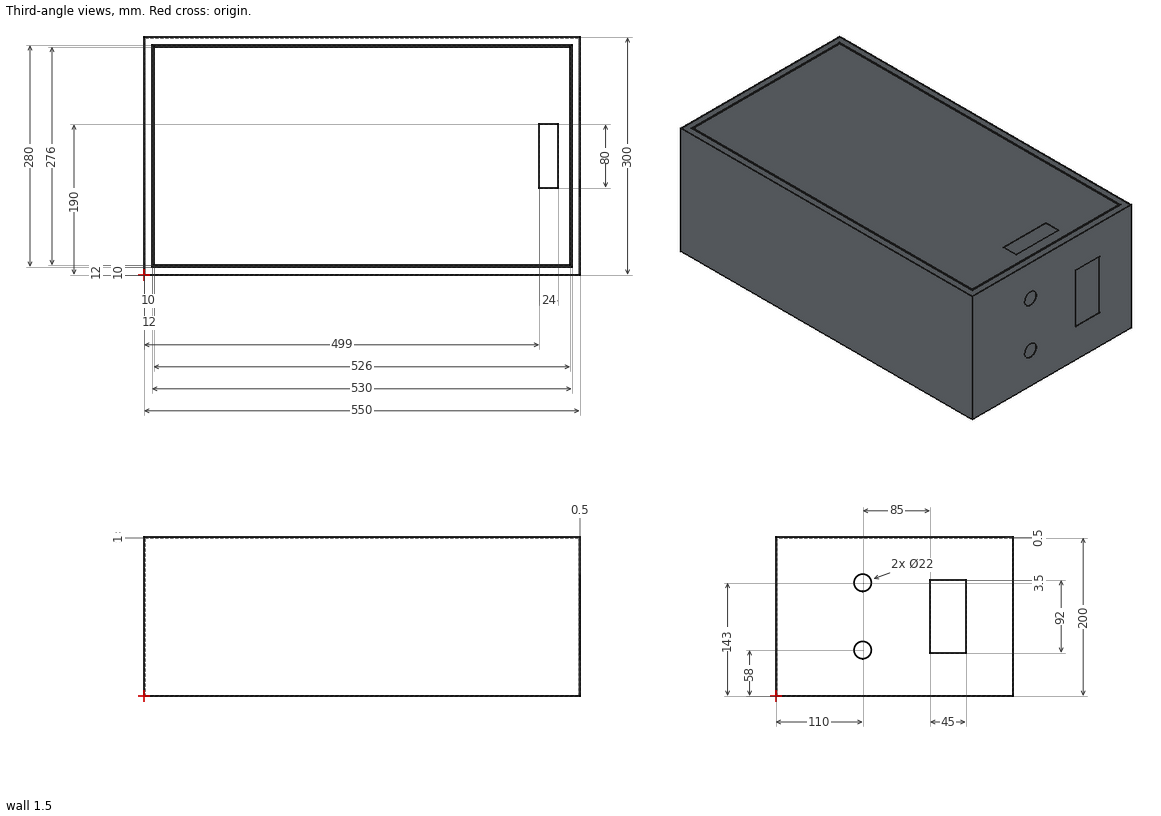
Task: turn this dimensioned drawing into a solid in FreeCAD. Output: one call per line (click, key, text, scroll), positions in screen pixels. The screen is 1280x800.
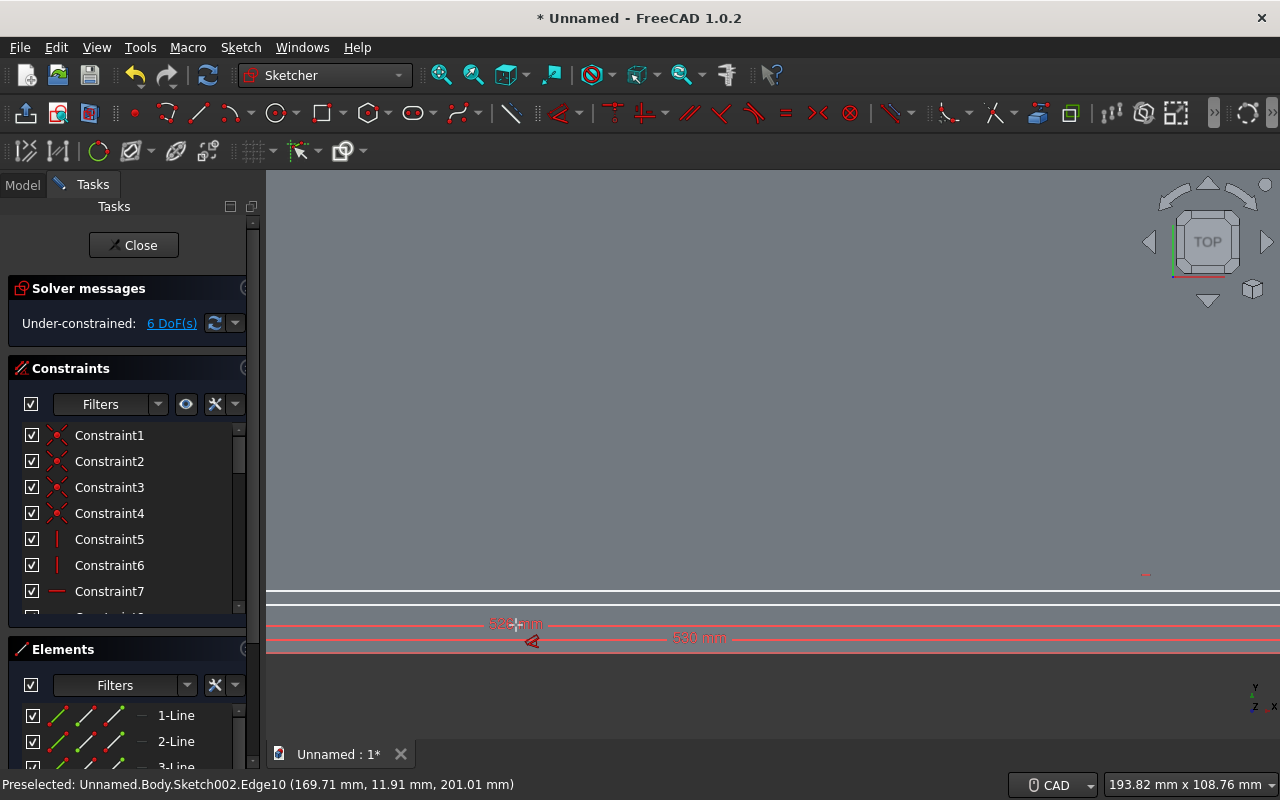
scroll(599, 596, down, 8)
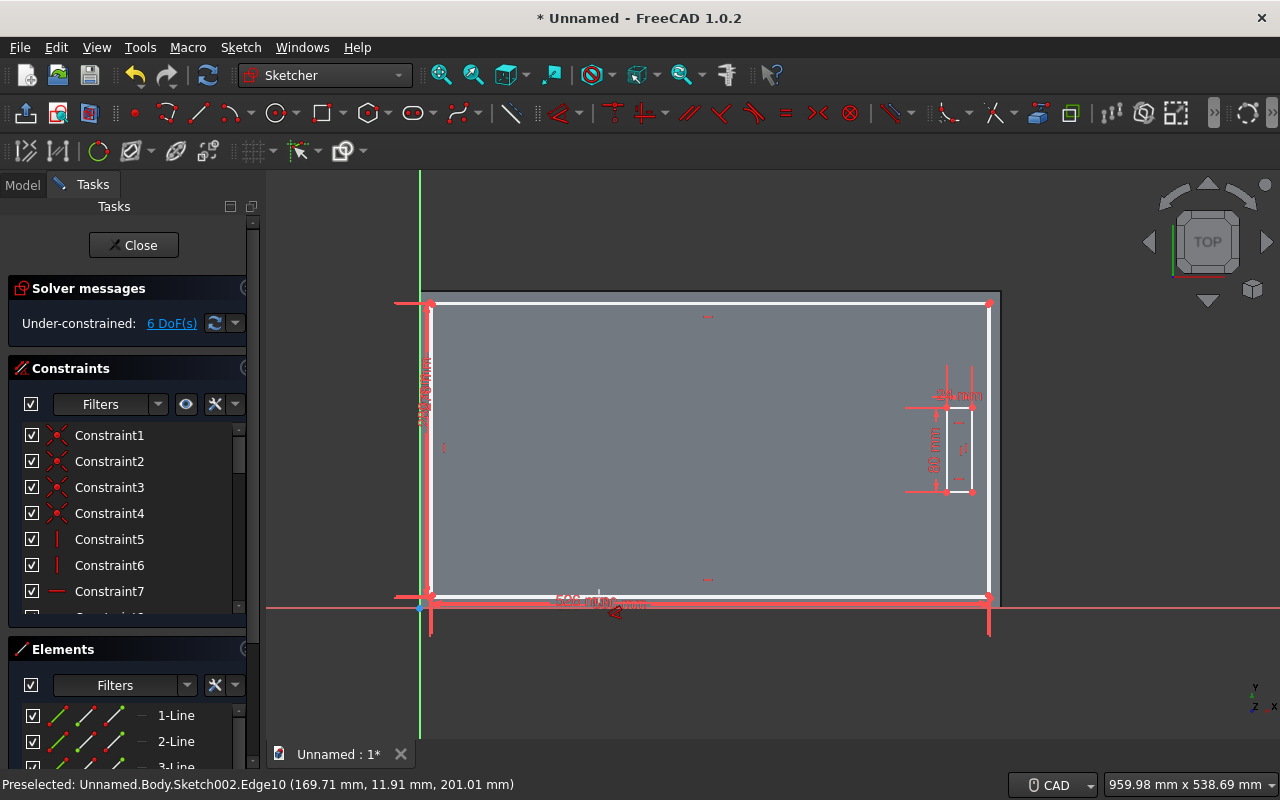
scroll(430, 303, up, 8)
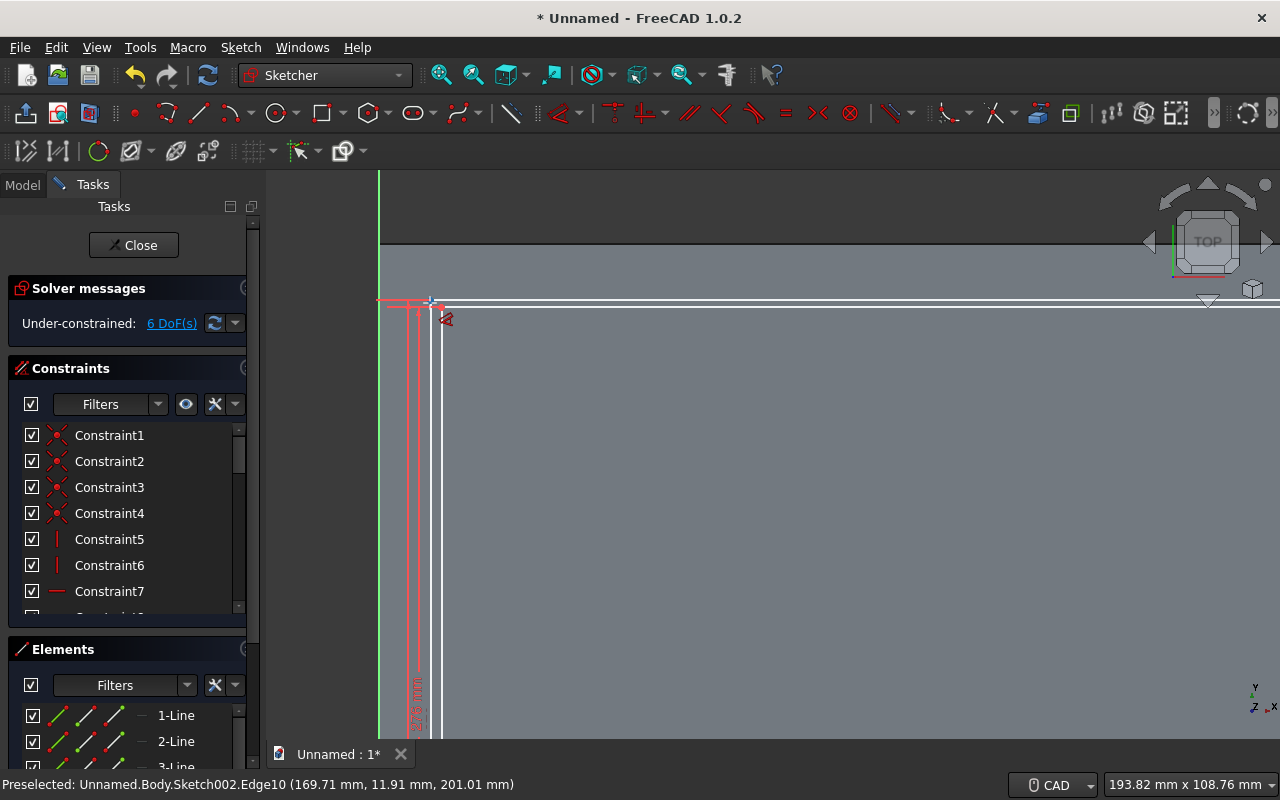
click(431, 300)
click(405, 266)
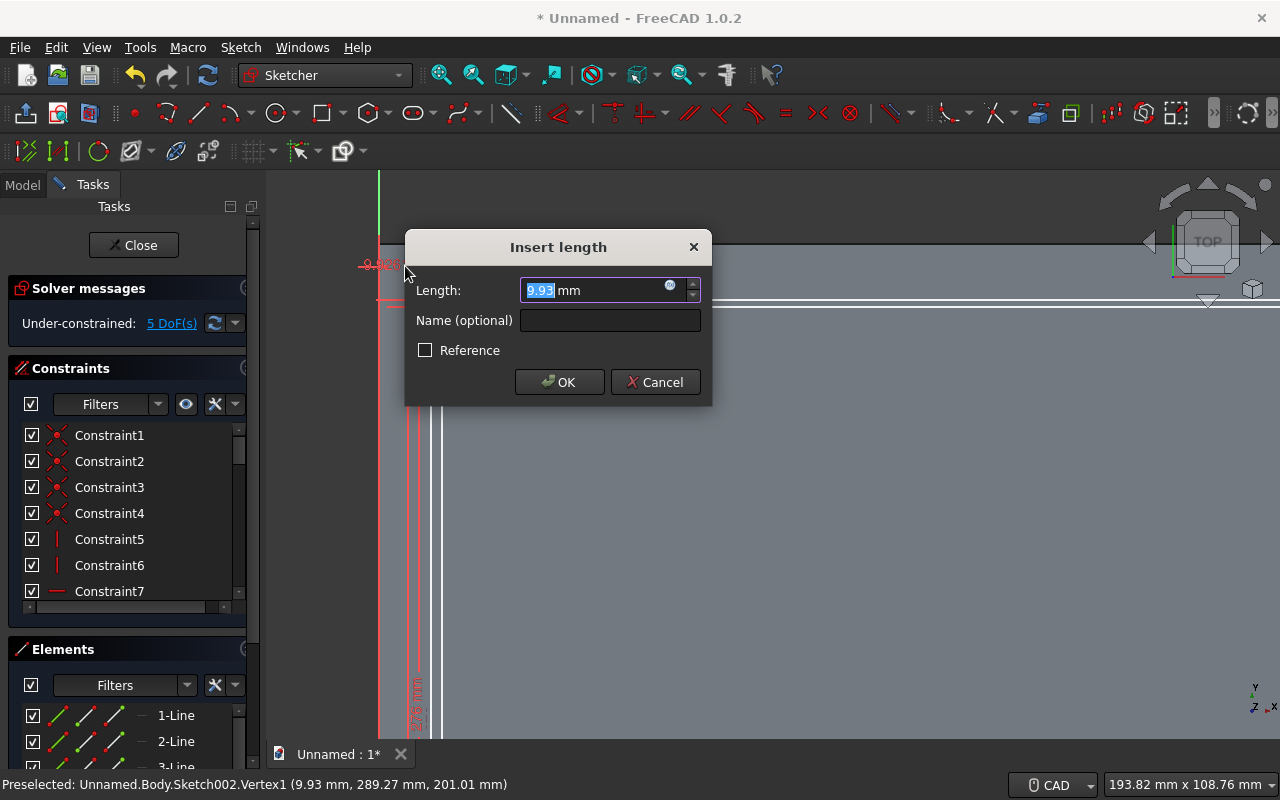
text(10)
key(Return)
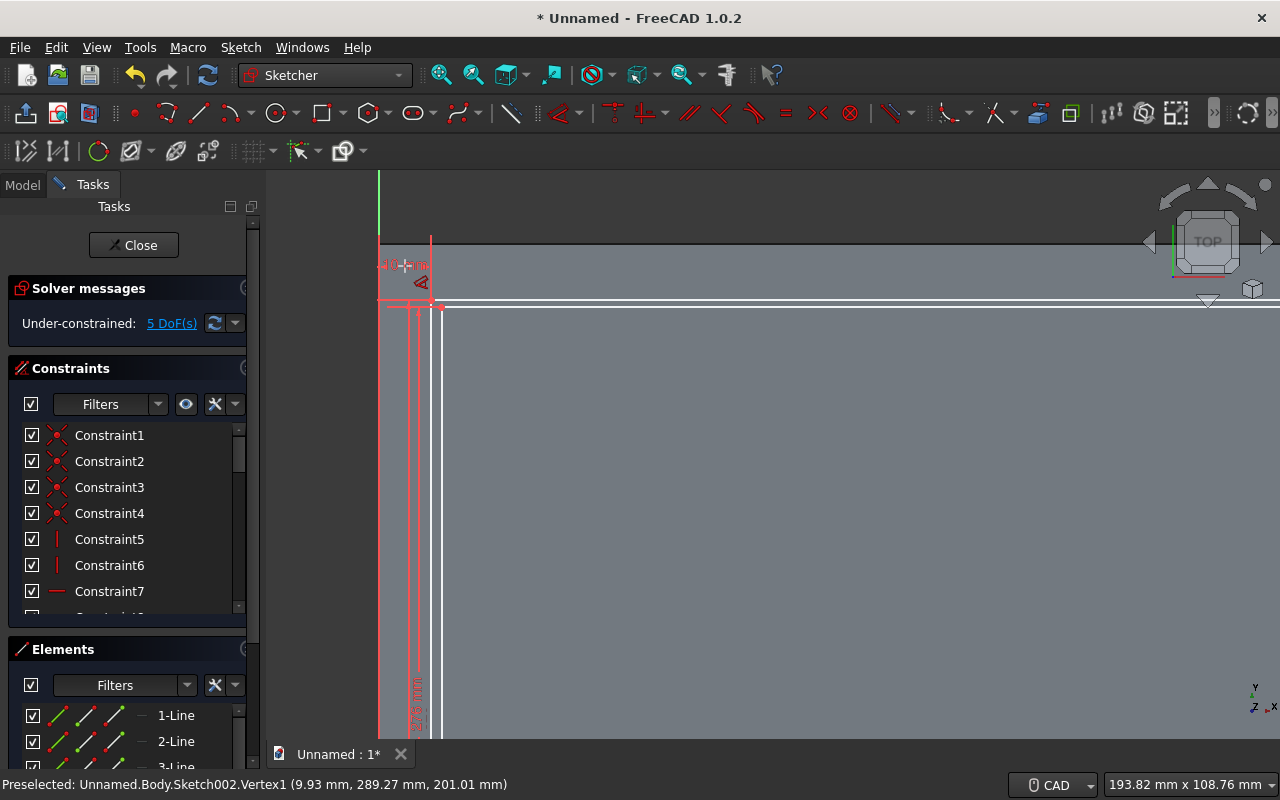
scroll(430, 303, down, 8)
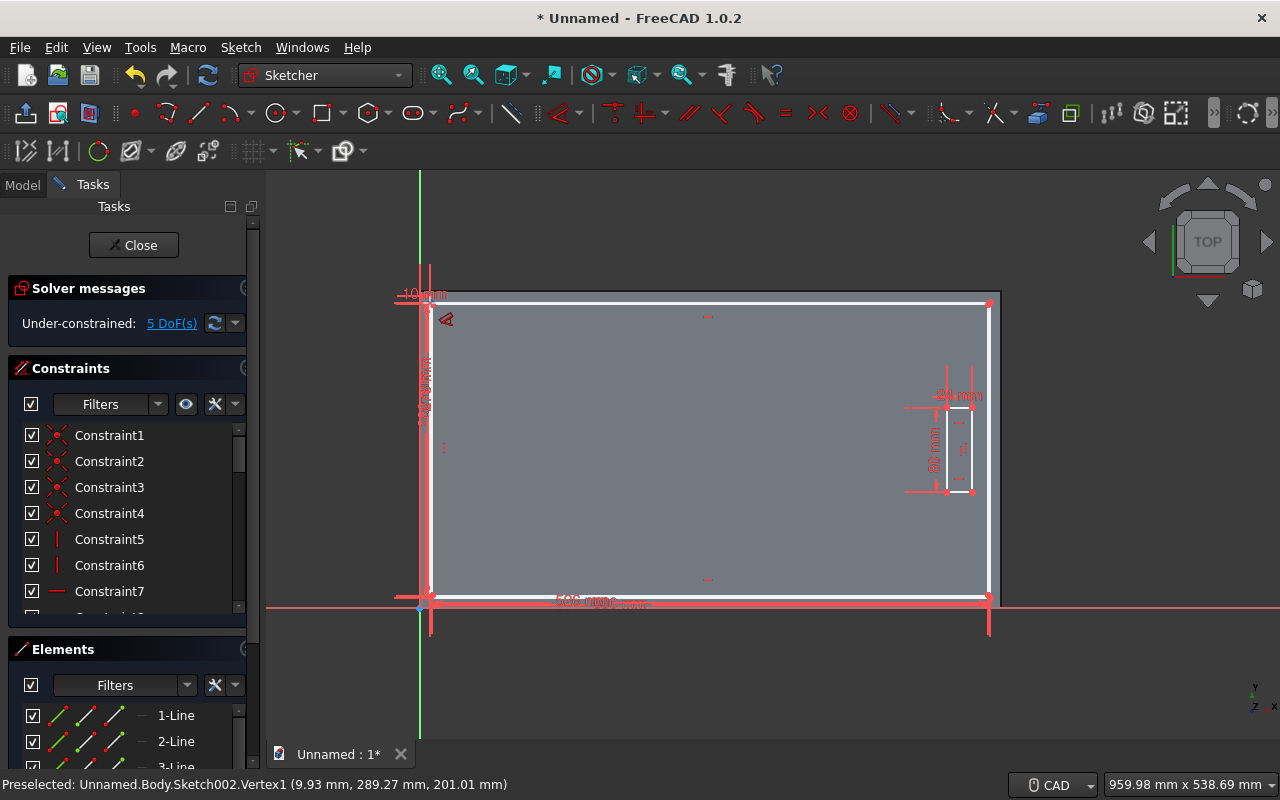
scroll(430, 598, up, 7)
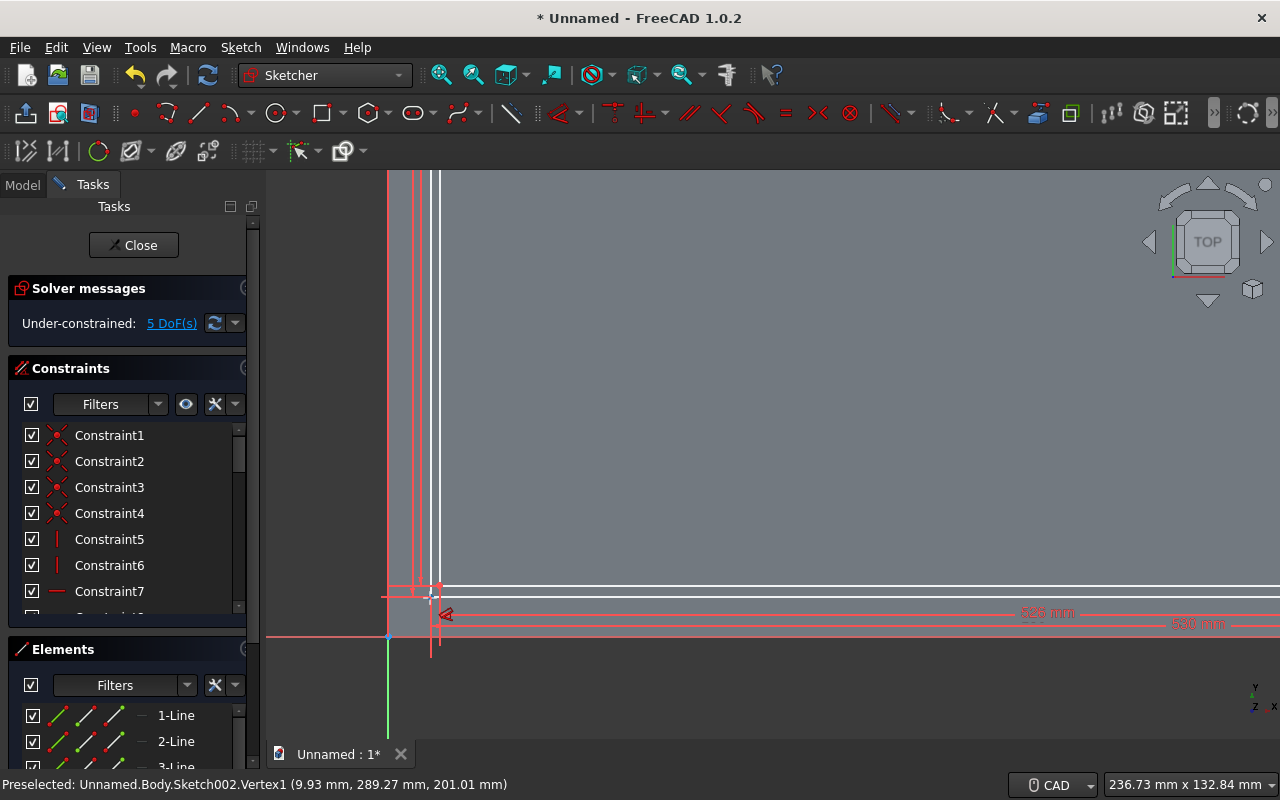
click(431, 597)
click(354, 617)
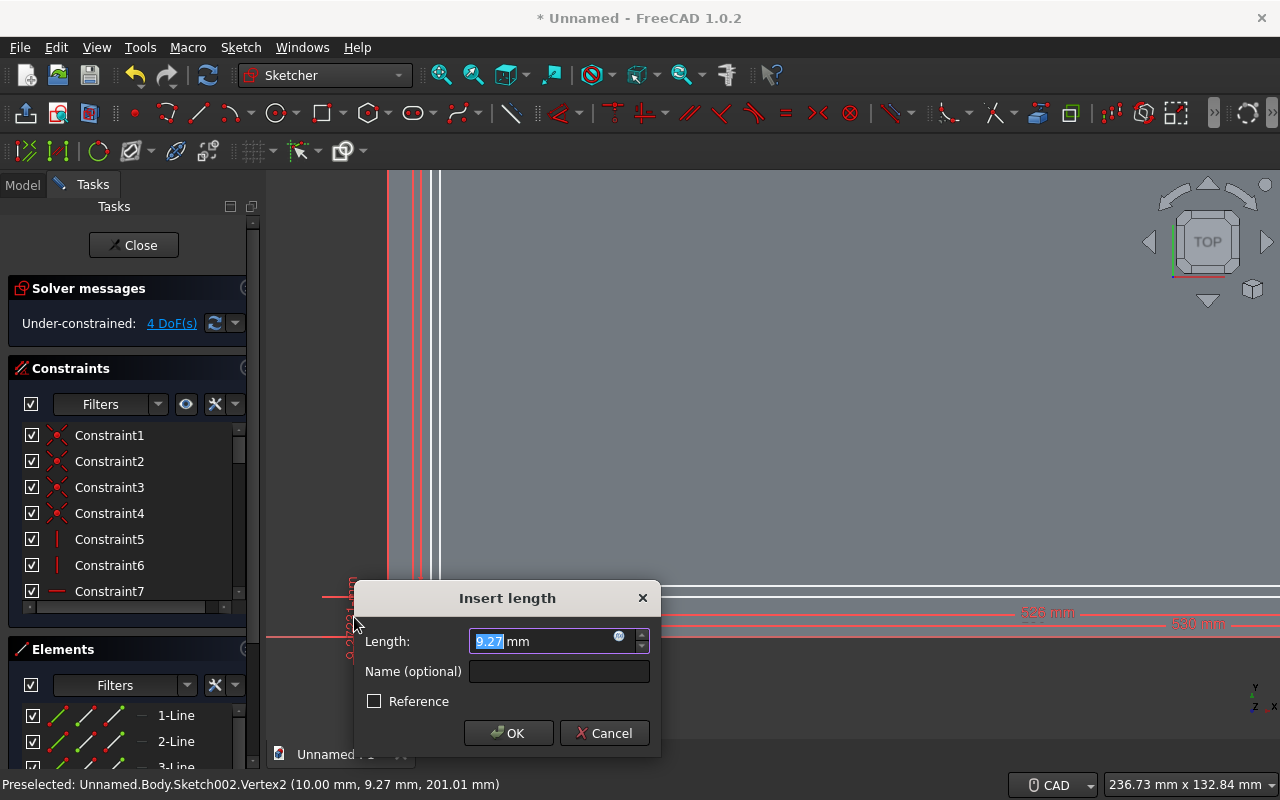
text(10)
key(Return)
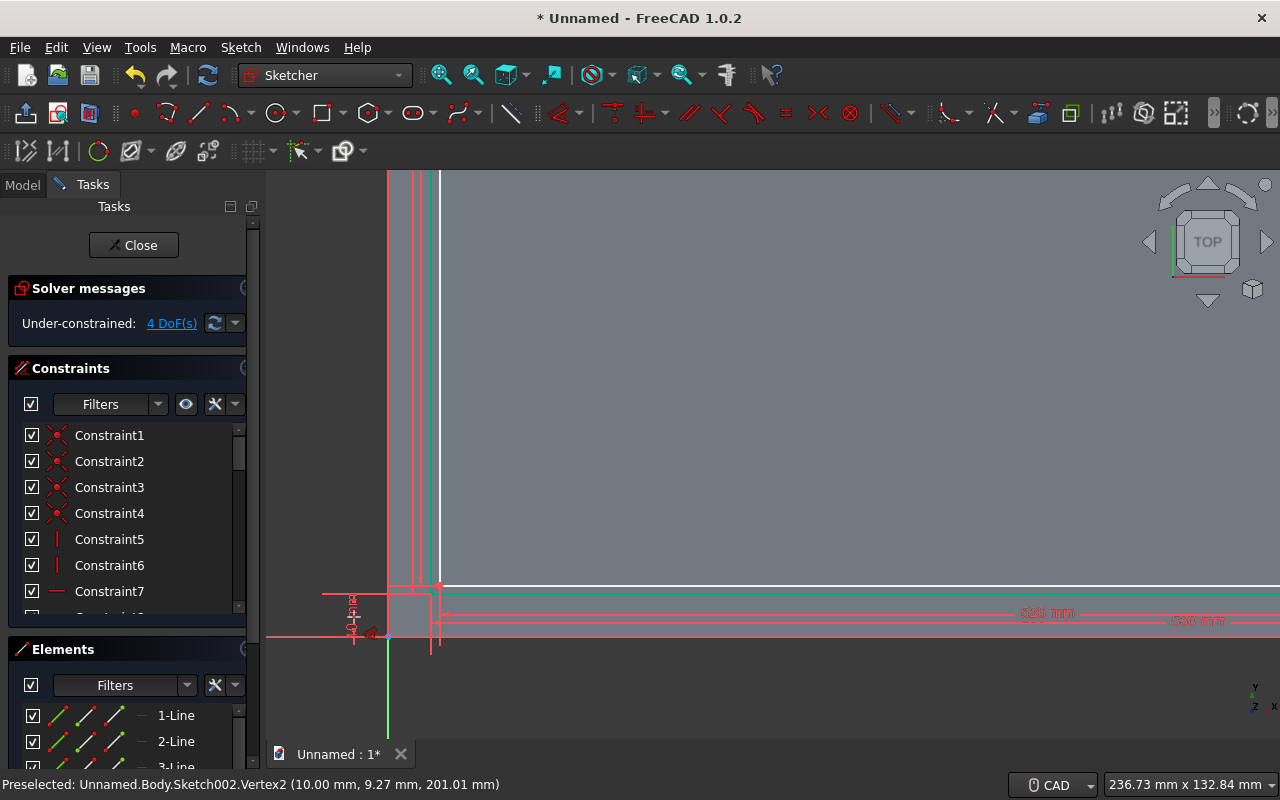
scroll(430, 598, down, 7)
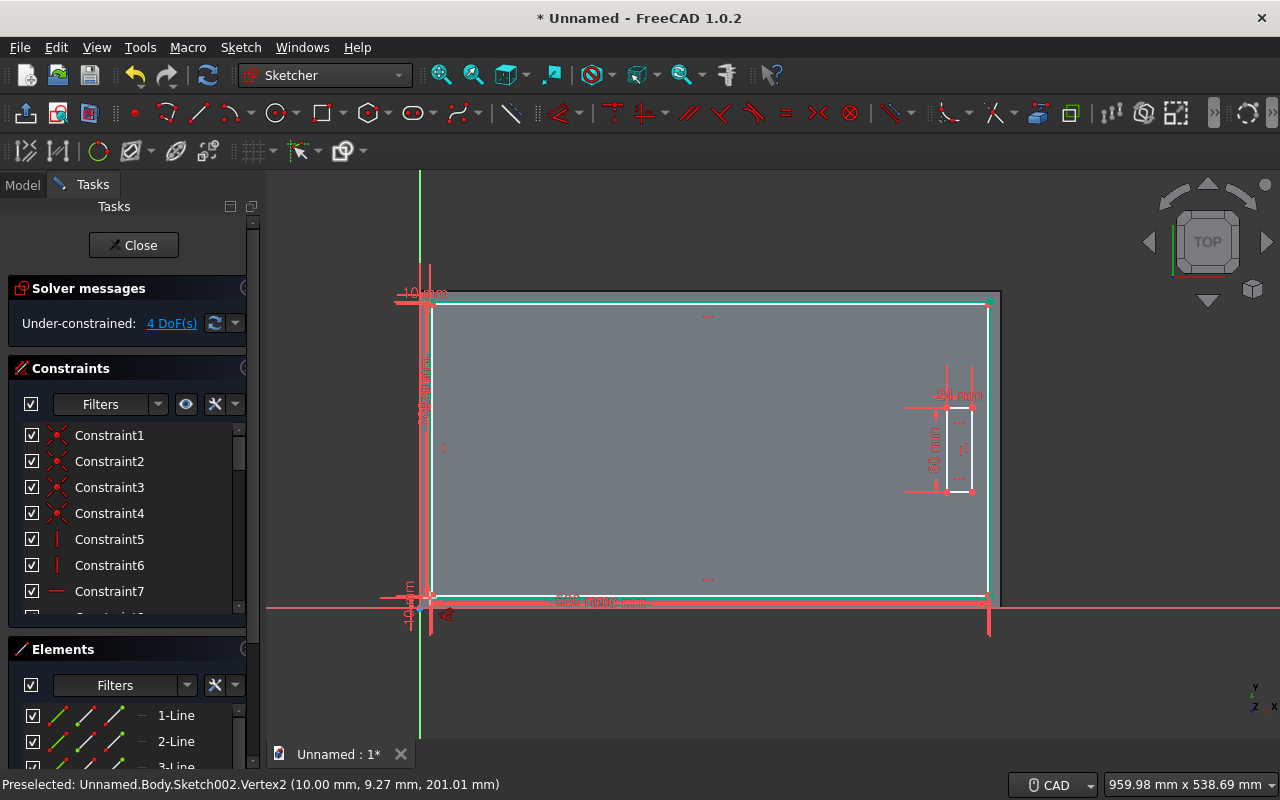
scroll(432, 304, up, 7)